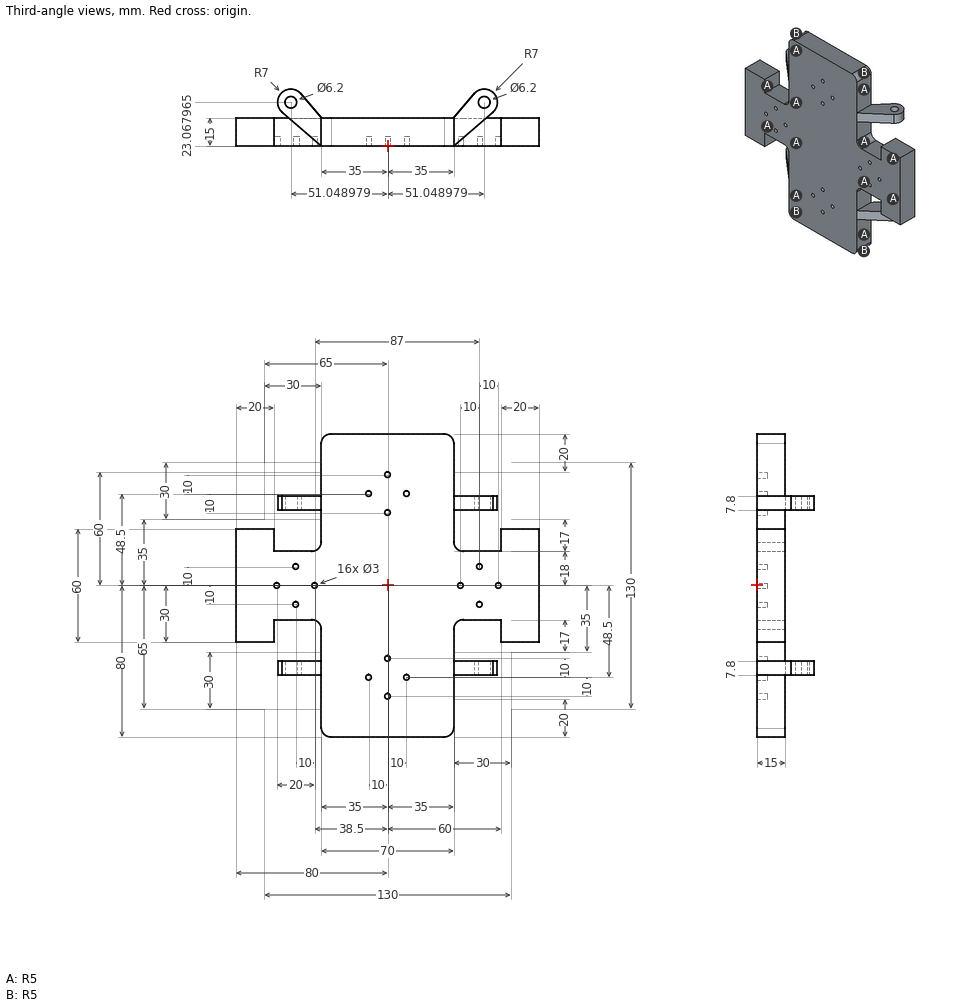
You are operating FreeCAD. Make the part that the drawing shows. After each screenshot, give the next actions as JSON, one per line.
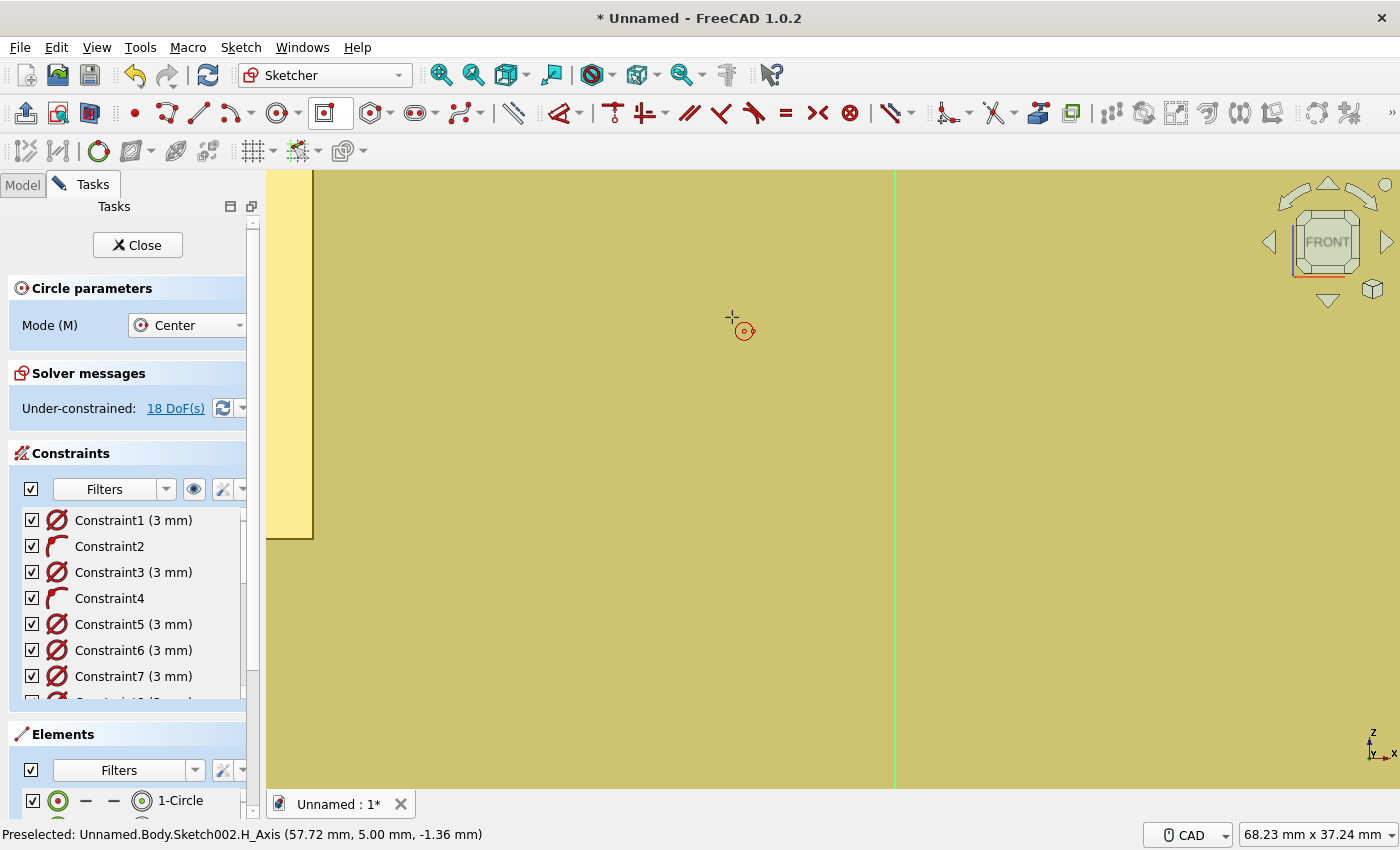
{"action": "scroll", "coordinate": [732, 317], "scroll_direction": "down", "scroll_amount": 8}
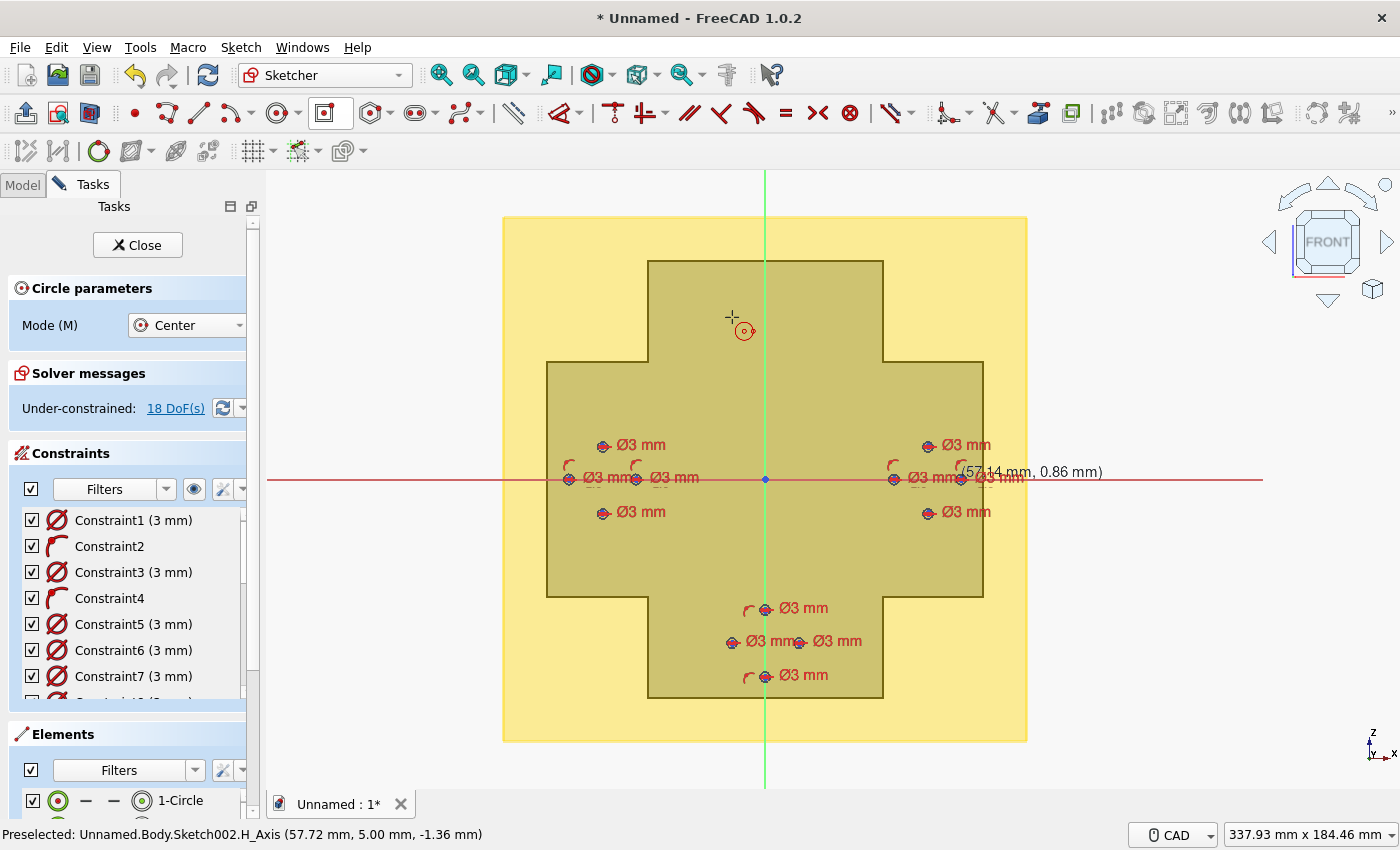
{"action": "left_click", "coordinate": [732, 317]}
{"action": "mouse_move", "coordinate": [735, 313]}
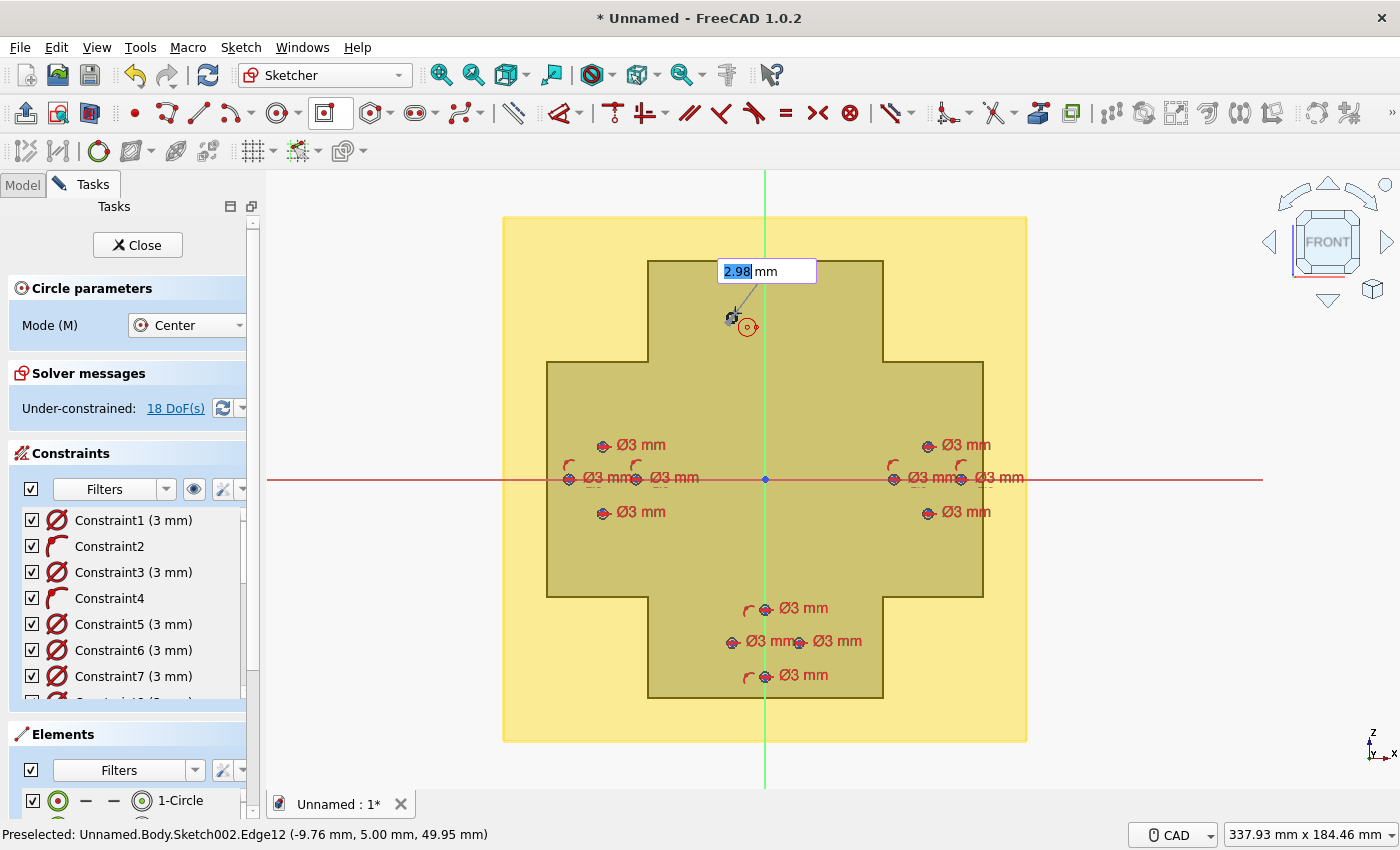
{"action": "type", "text": "3"}
{"action": "key", "text": "Return"}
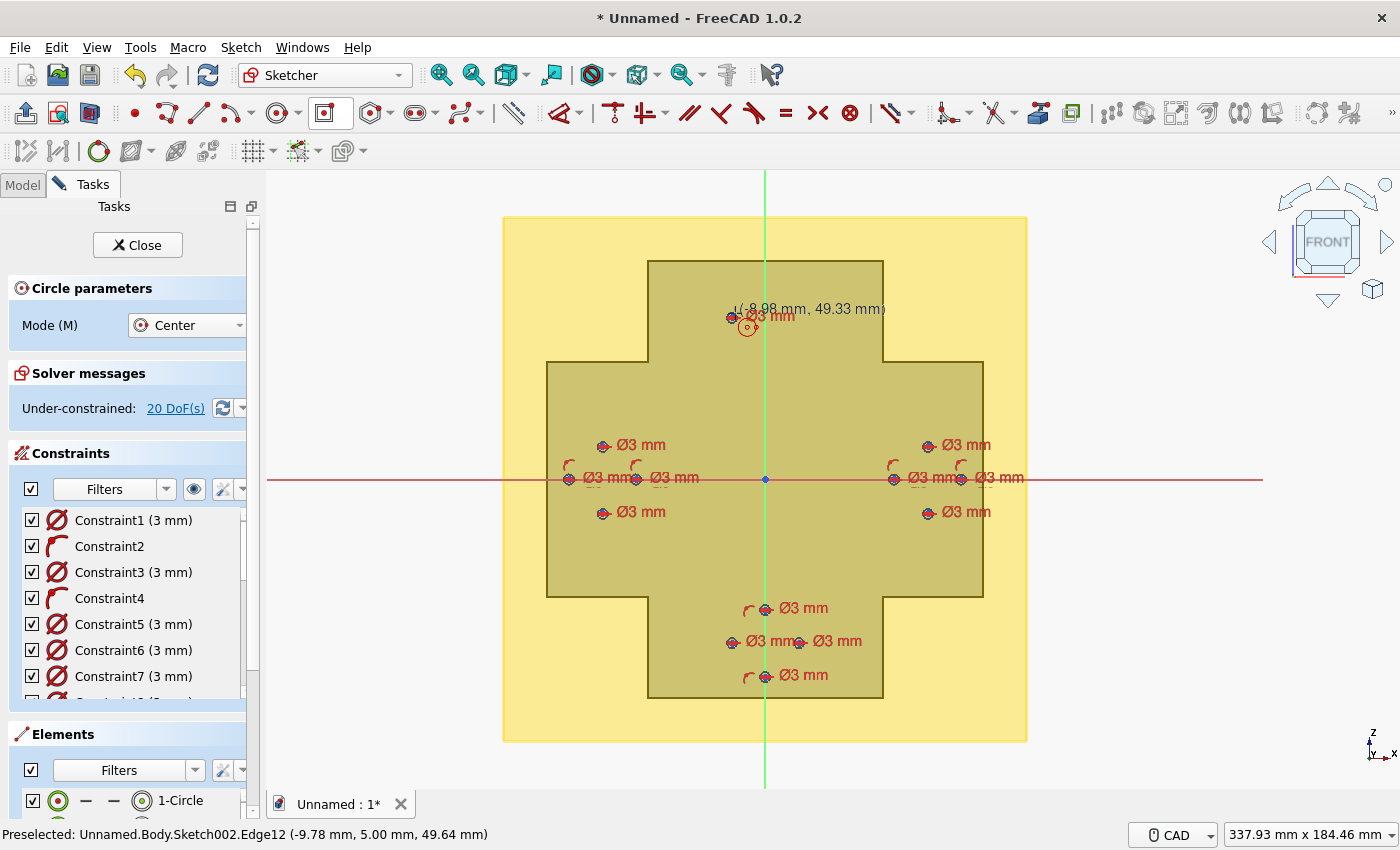
{"action": "scroll", "coordinate": [765, 350], "scroll_direction": "up", "scroll_amount": 8}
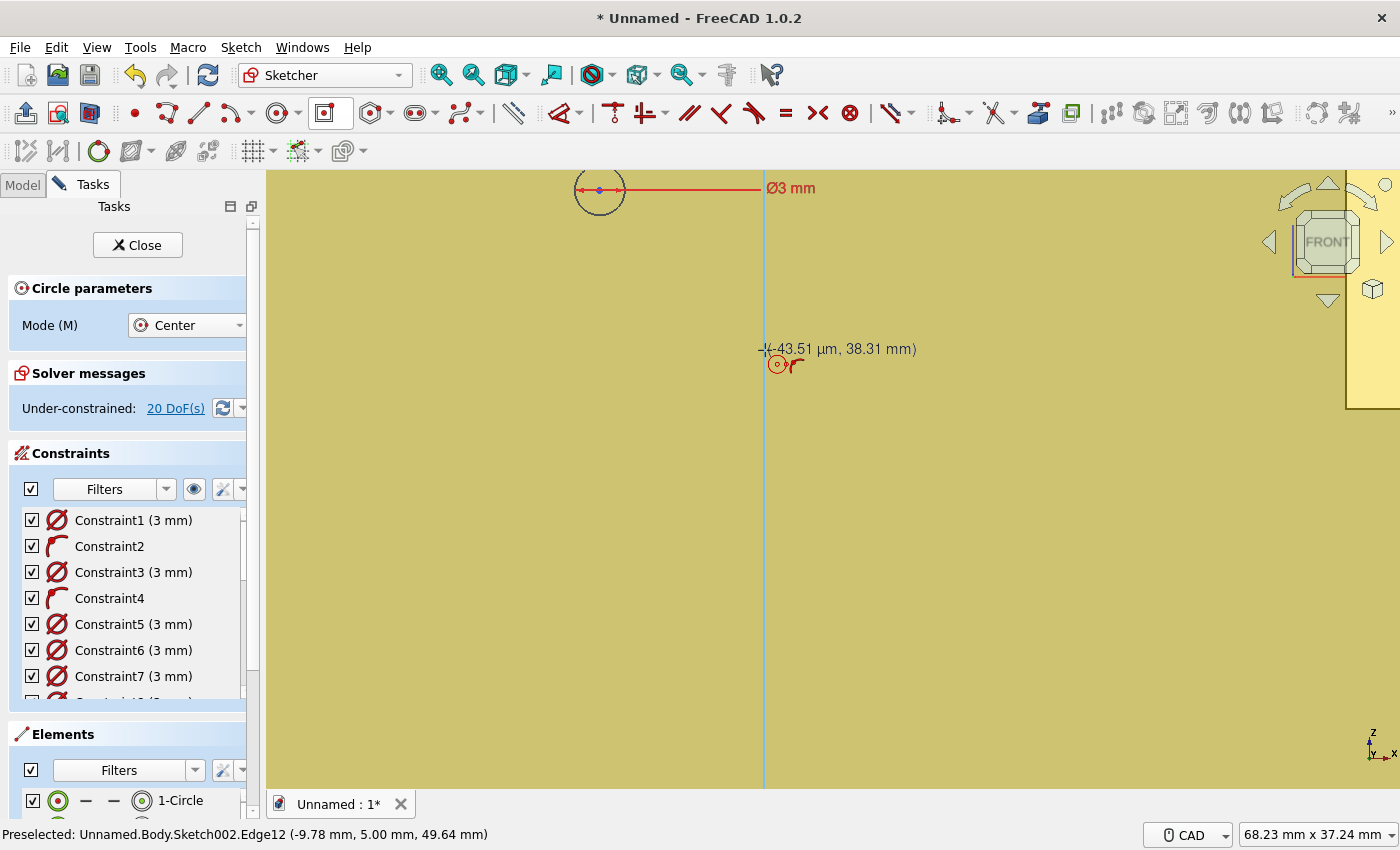
{"action": "scroll", "coordinate": [765, 350], "scroll_direction": "down", "scroll_amount": 8}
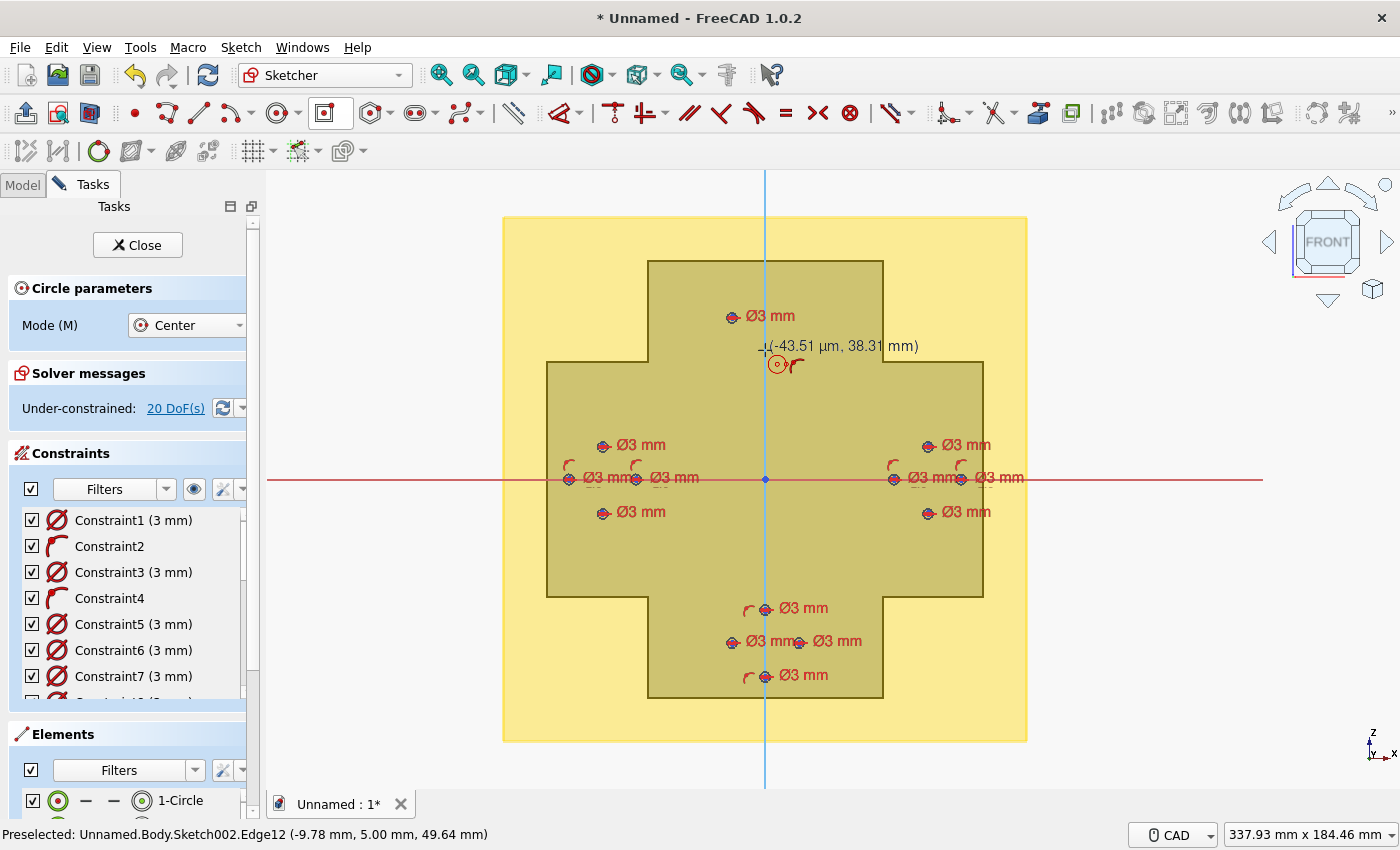
{"action": "left_click", "coordinate": [765, 350]}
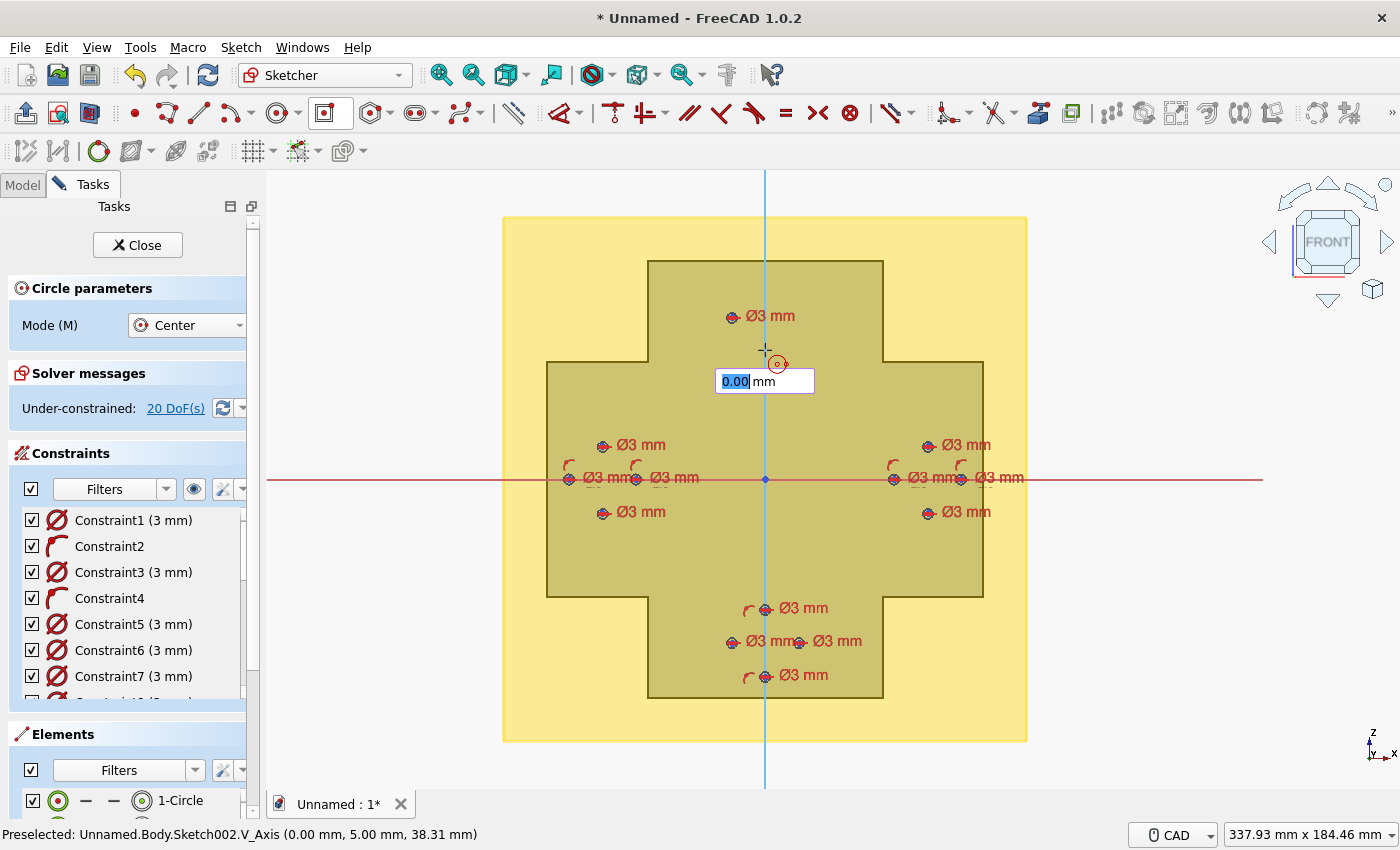
{"action": "scroll", "coordinate": [770, 349], "scroll_direction": "up", "scroll_amount": 7}
{"action": "mouse_move", "coordinate": [768, 347]}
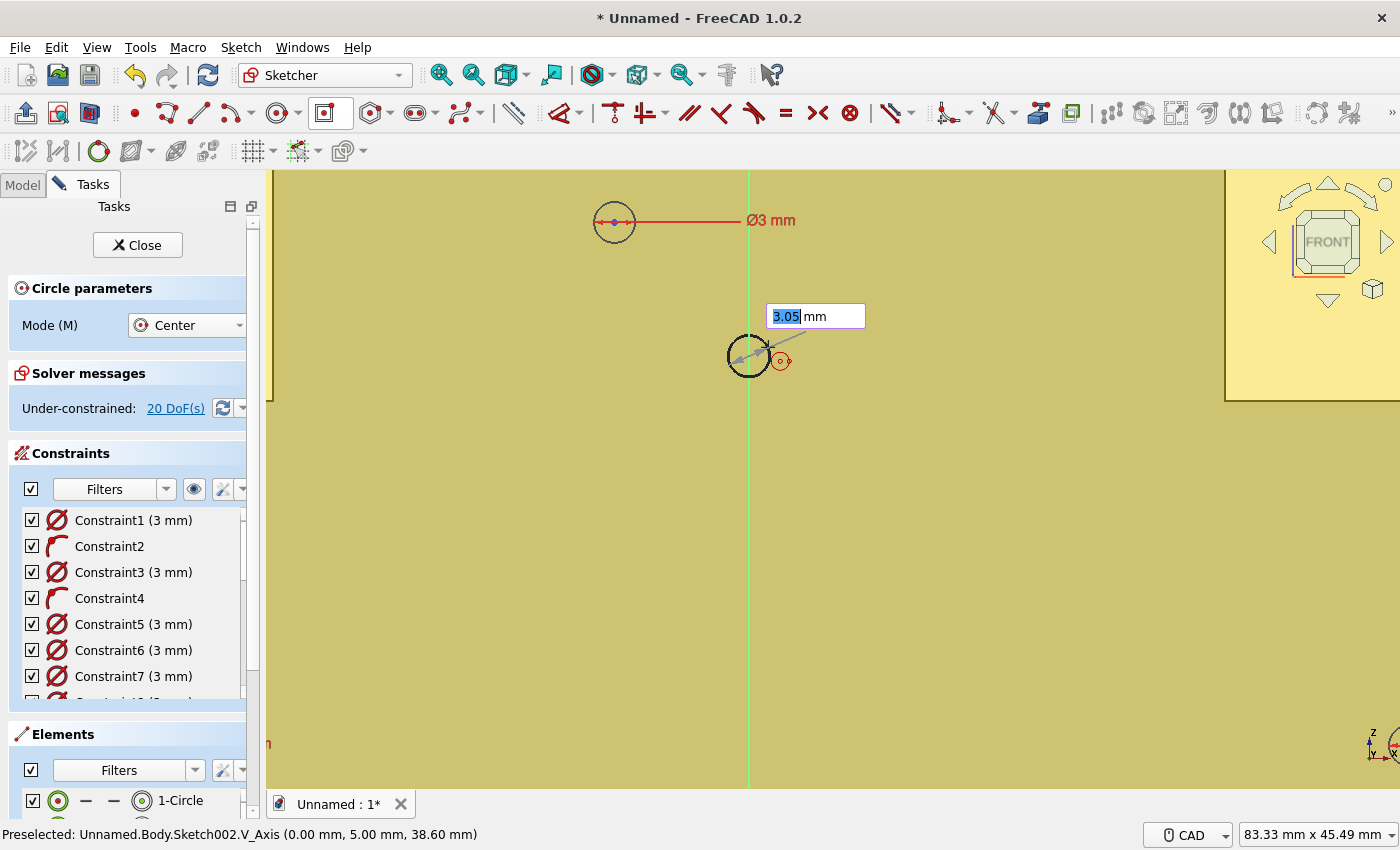
{"action": "type", "text": "3"}
{"action": "key", "text": "Return"}